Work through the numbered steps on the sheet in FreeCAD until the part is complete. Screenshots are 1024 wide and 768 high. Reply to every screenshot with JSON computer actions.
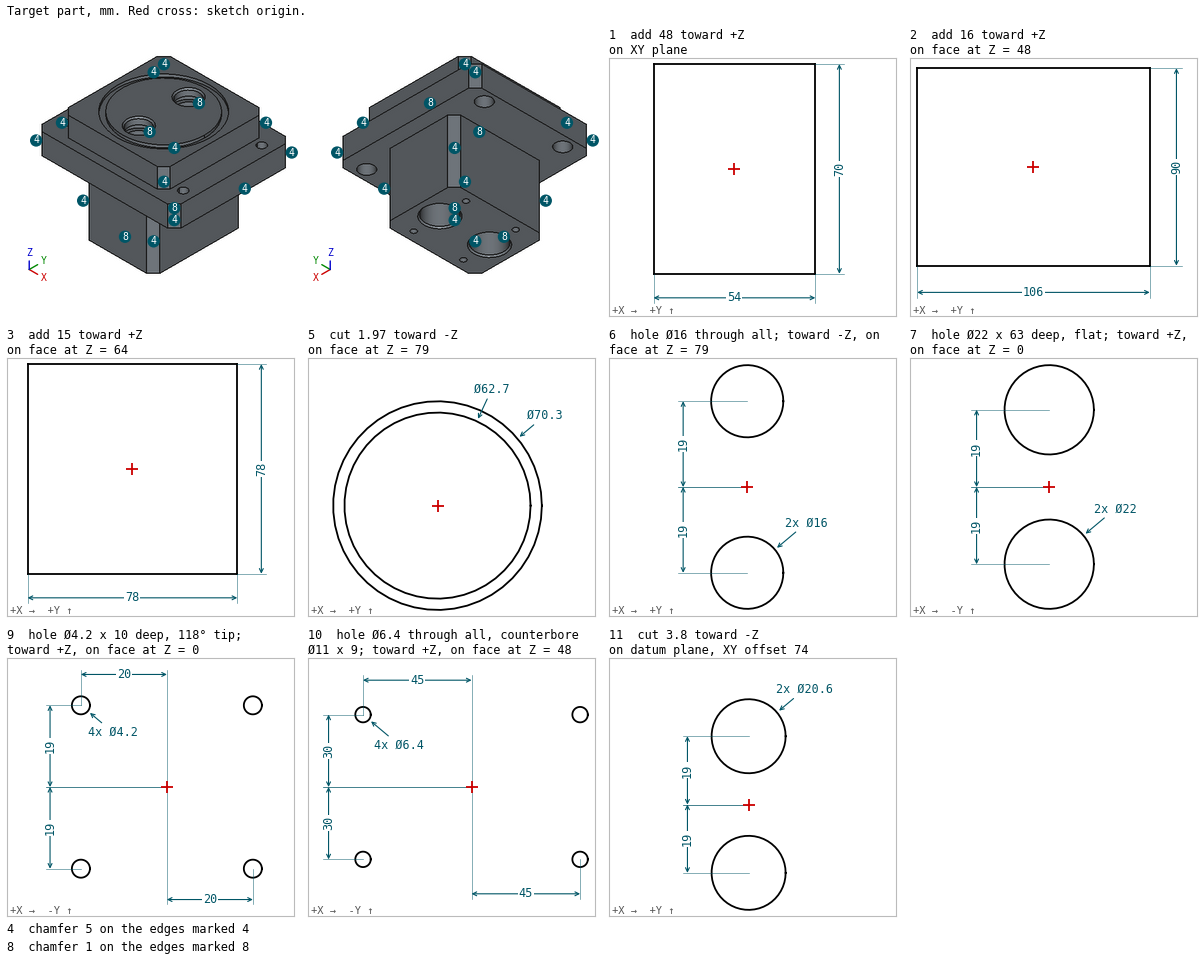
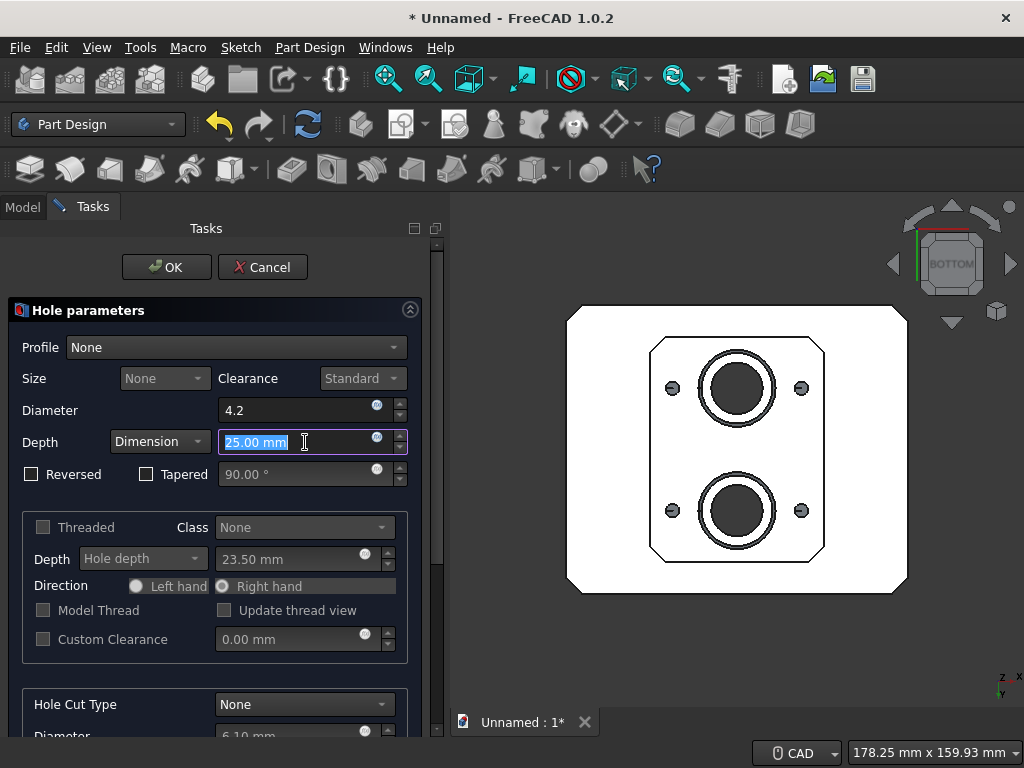
{"action": "type", "text": "10"}
{"action": "key", "text": "Tab"}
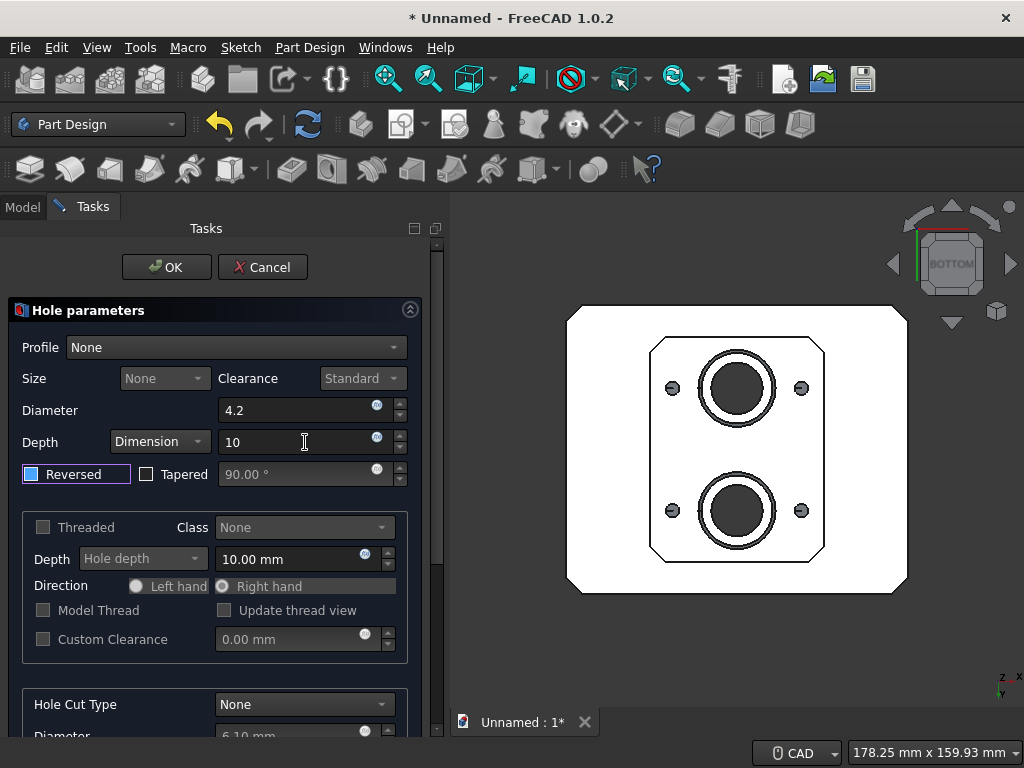
{"action": "left_click", "coordinate": [167, 267]}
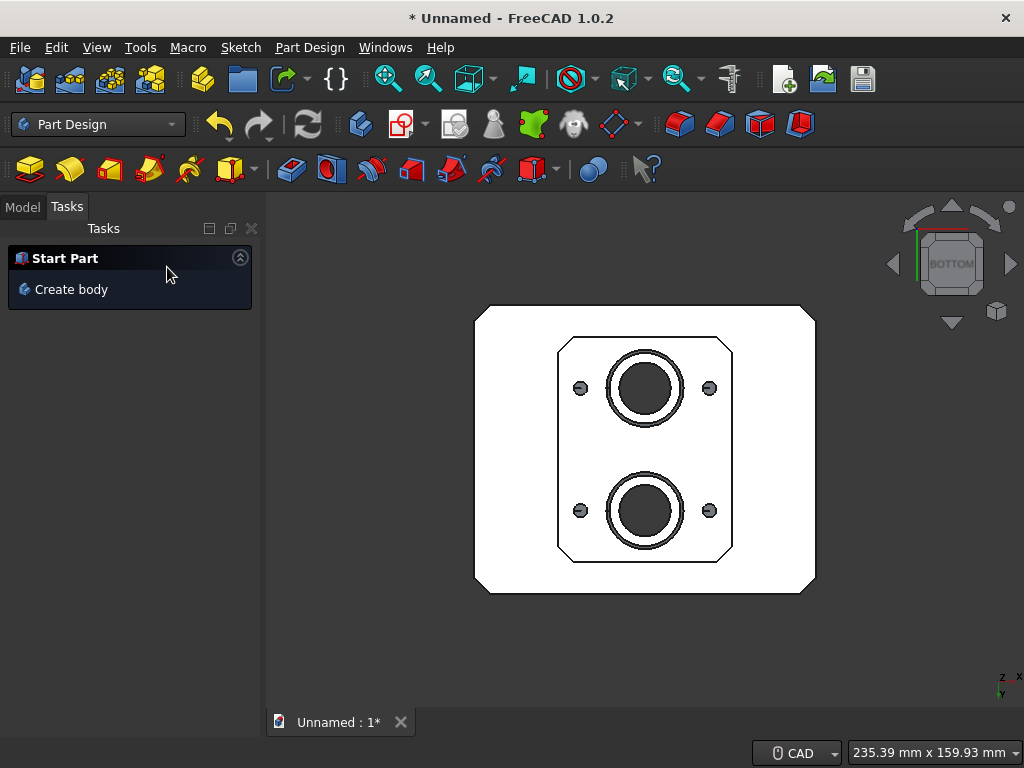
{"action": "left_click", "coordinate": [791, 531]}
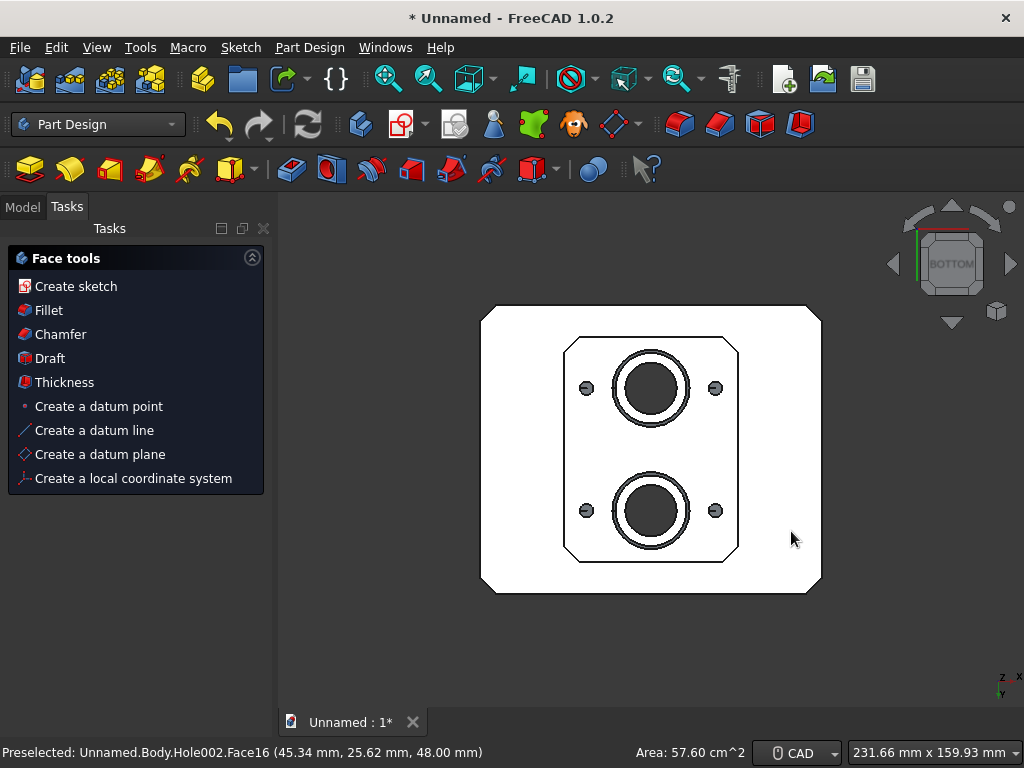
{"action": "left_click", "coordinate": [402, 124]}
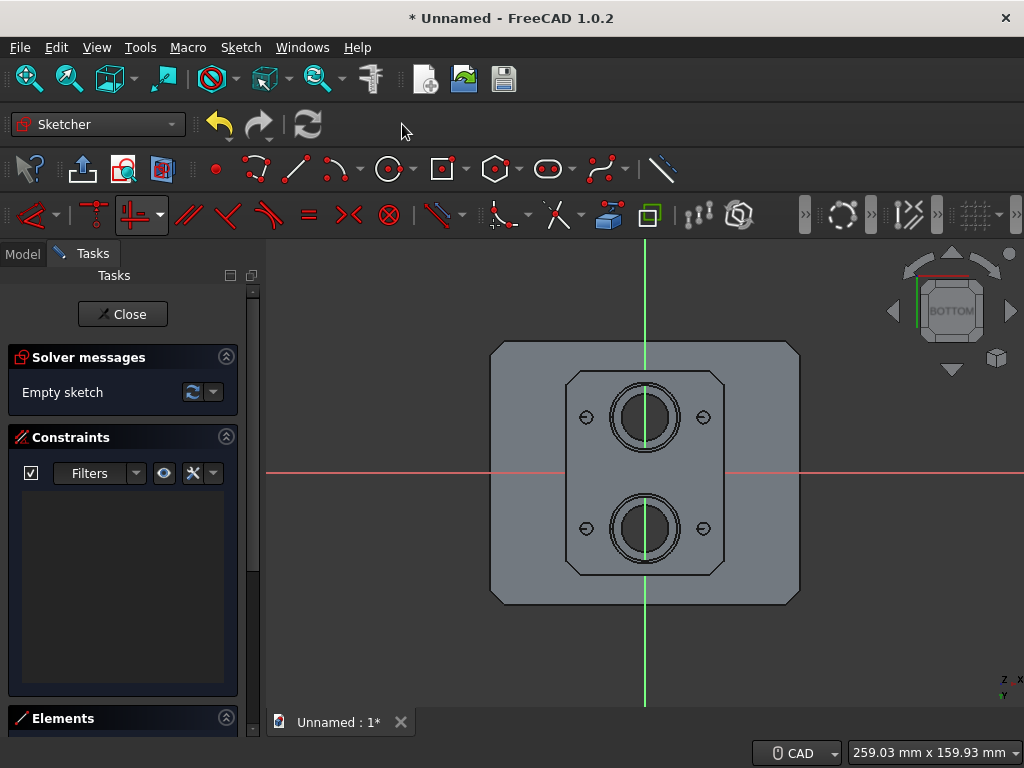
{"action": "scroll", "coordinate": [784, 473], "scroll_direction": "up", "scroll_amount": 2}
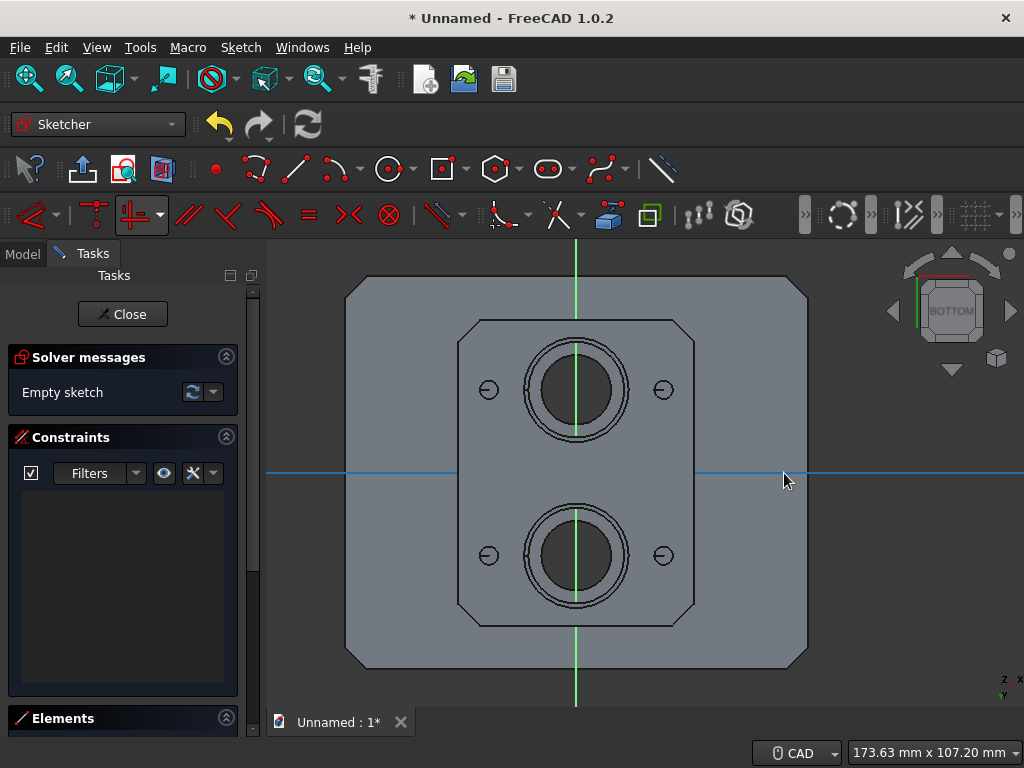
{"action": "left_click", "coordinate": [390, 170]}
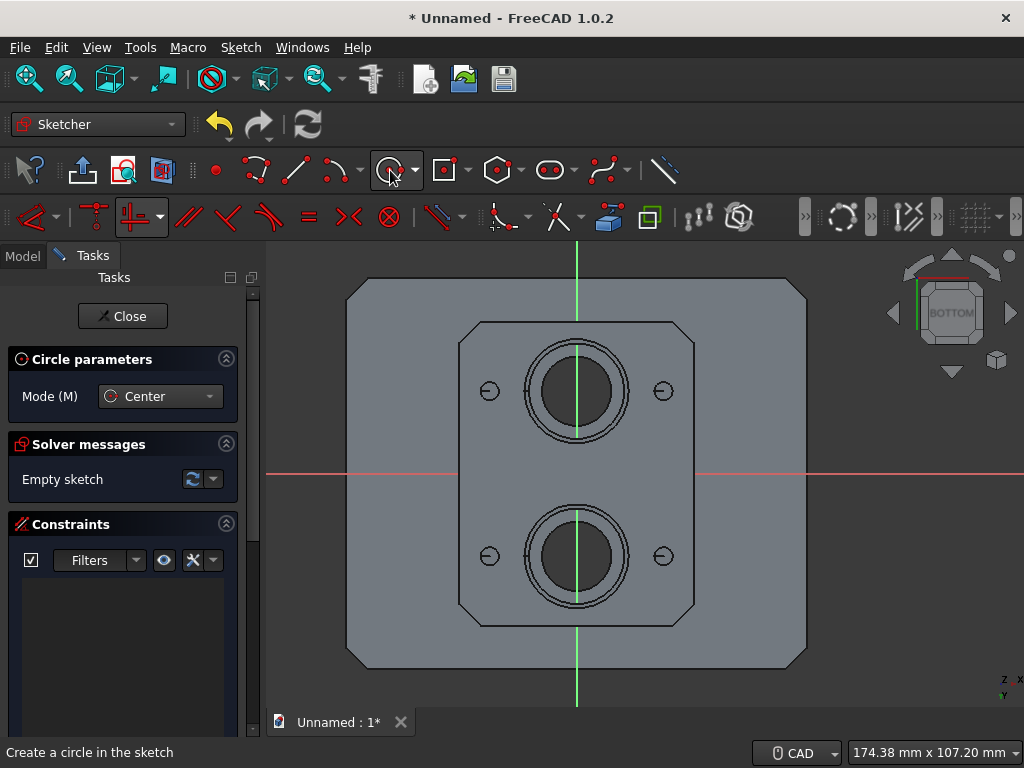
{"action": "scroll", "coordinate": [381, 343], "scroll_direction": "up", "scroll_amount": 3}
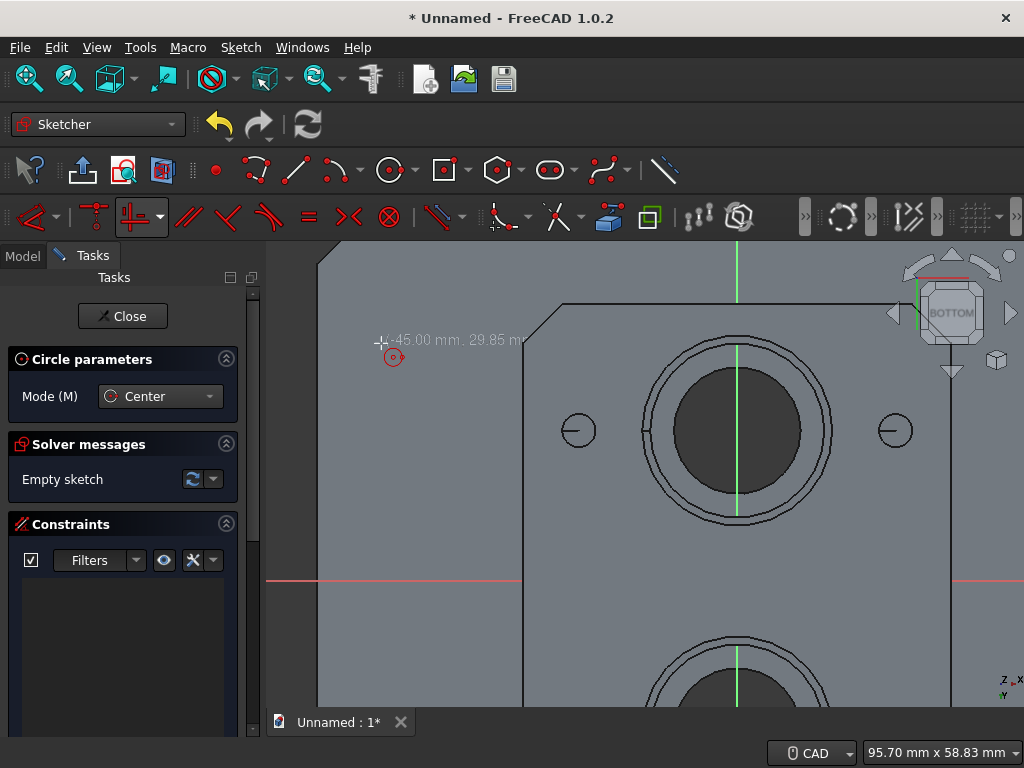
{"action": "left_click", "coordinate": [381, 343]}
{"action": "mouse_move", "coordinate": [399, 326]}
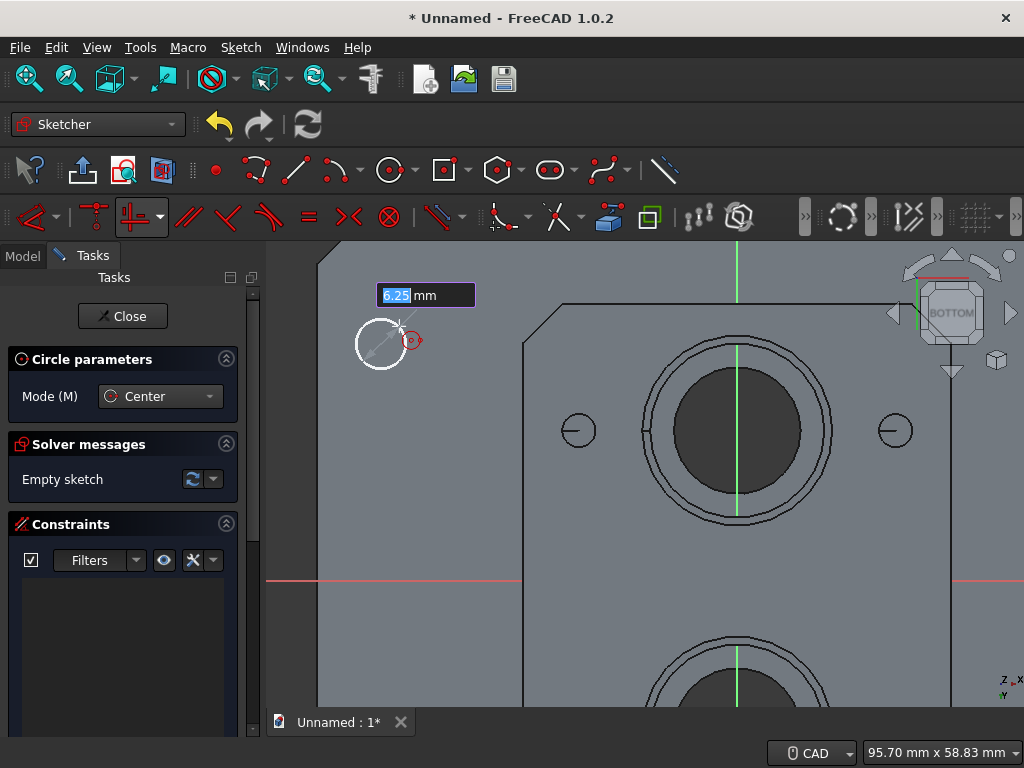
{"action": "type", "text": "6.4"}
{"action": "key", "text": "Return"}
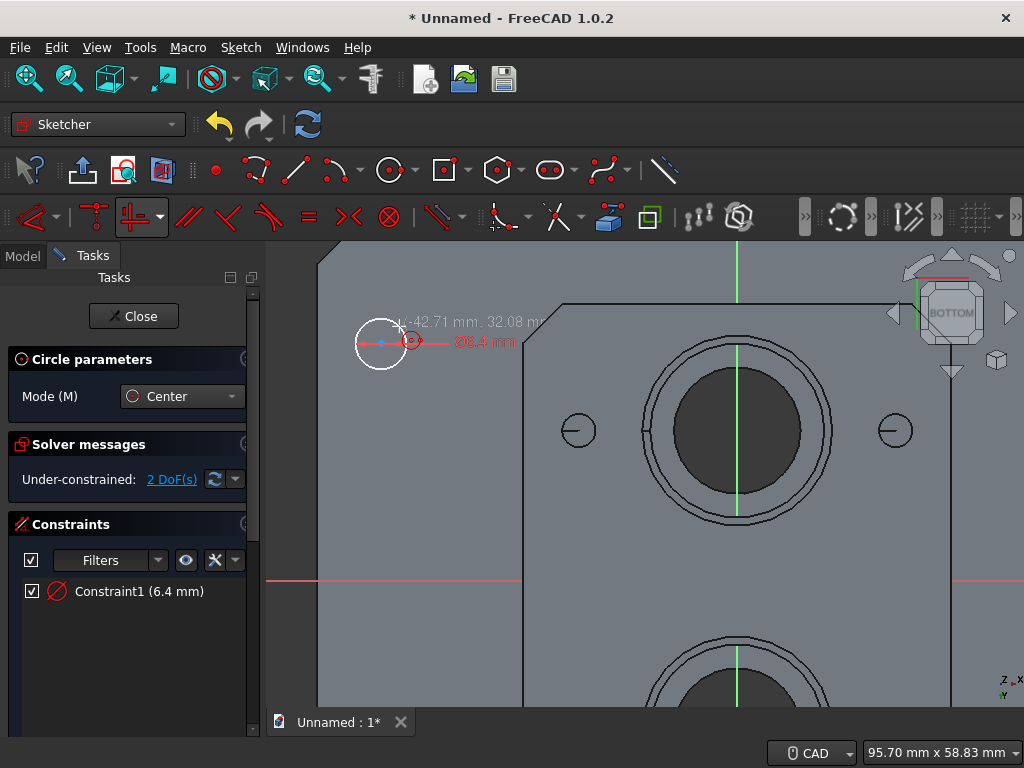
{"action": "scroll", "coordinate": [381, 344], "scroll_direction": "down", "scroll_amount": 3}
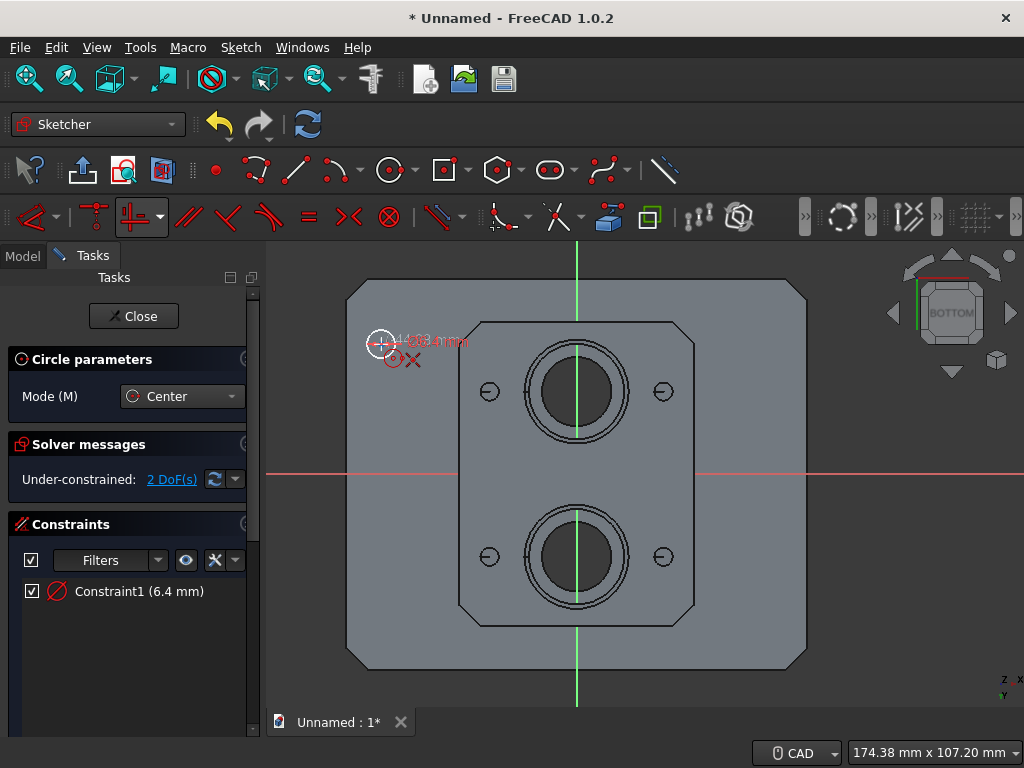
{"action": "scroll", "coordinate": [381, 605], "scroll_direction": "up", "scroll_amount": 3}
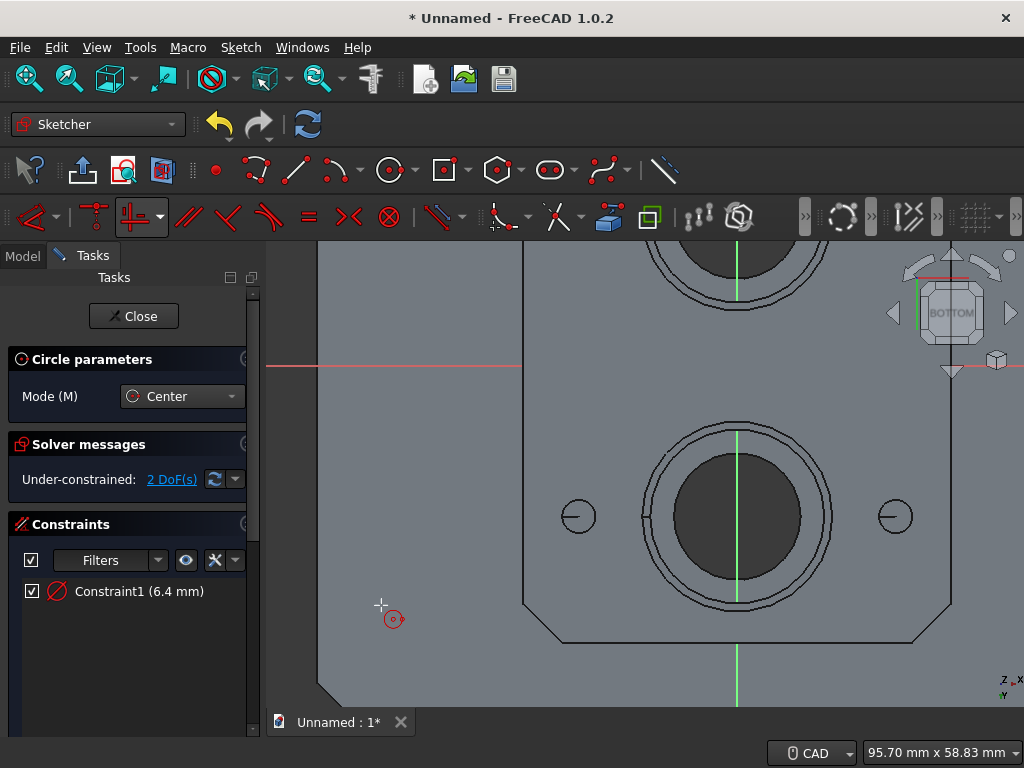
{"action": "left_click", "coordinate": [381, 604]}
{"action": "mouse_move", "coordinate": [399, 586]}